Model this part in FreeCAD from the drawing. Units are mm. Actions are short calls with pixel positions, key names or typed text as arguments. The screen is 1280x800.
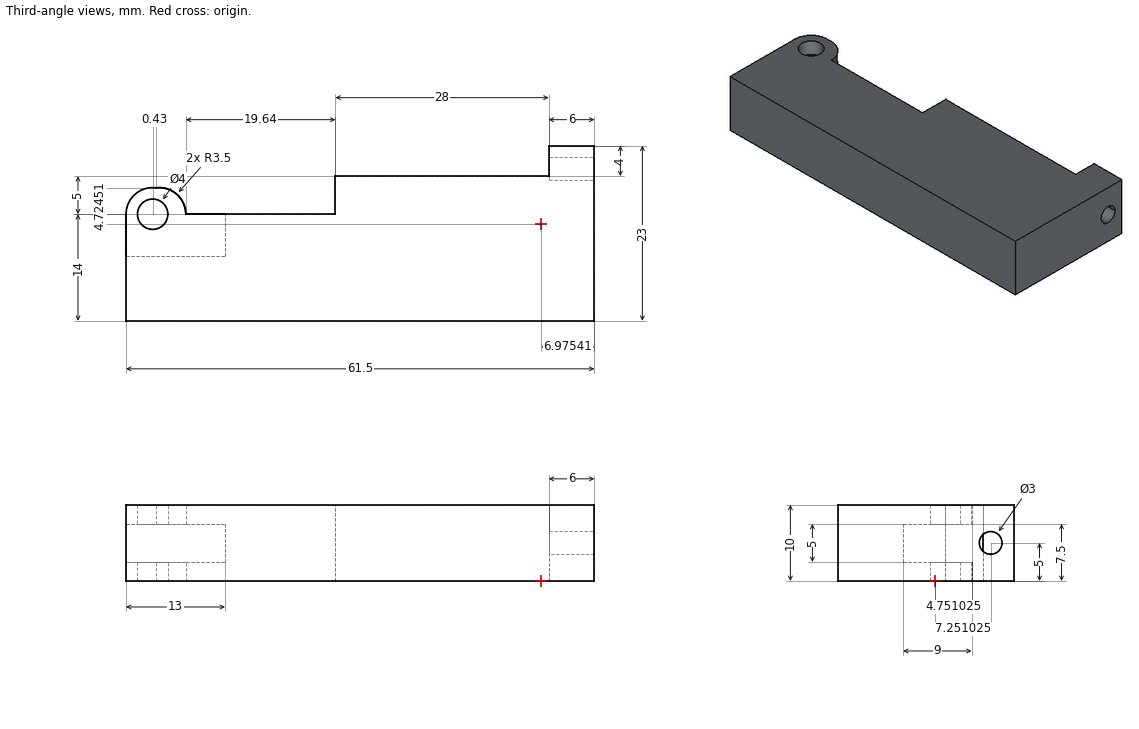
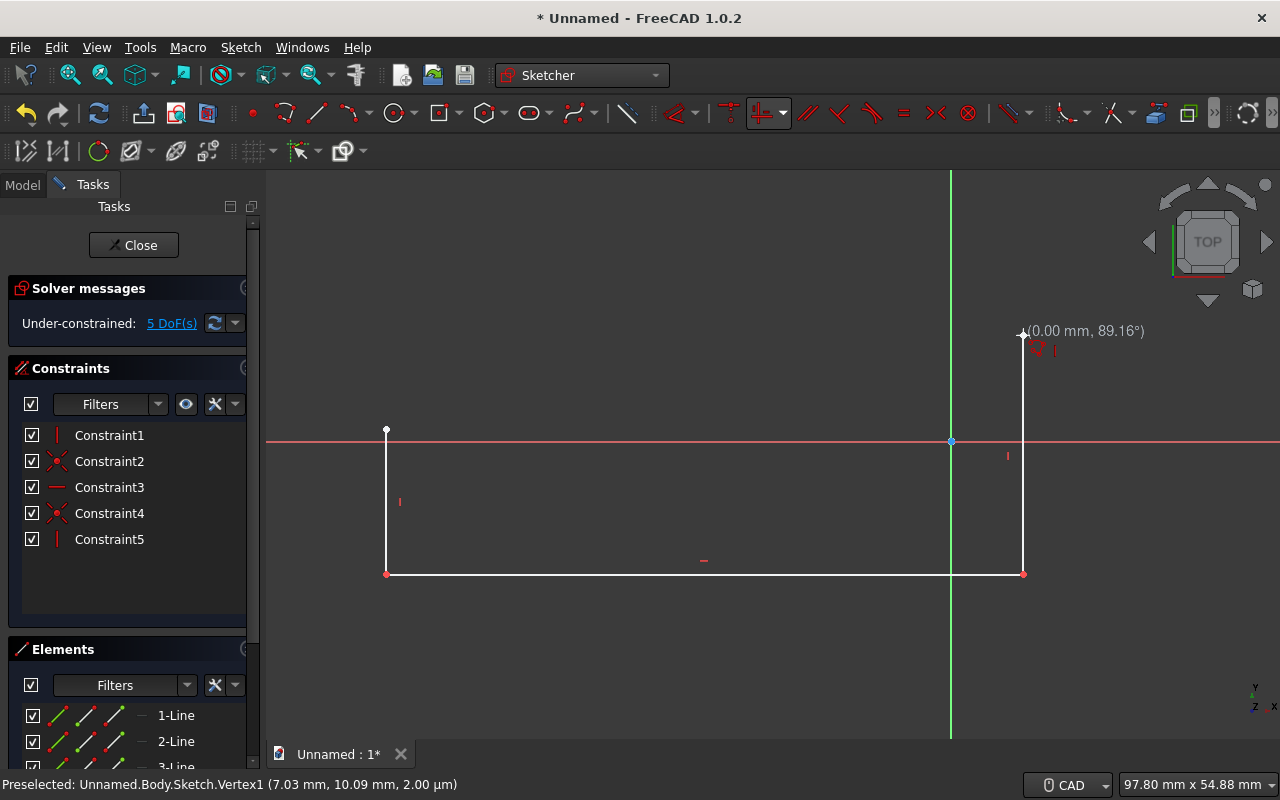
scroll(961, 335, up, 3)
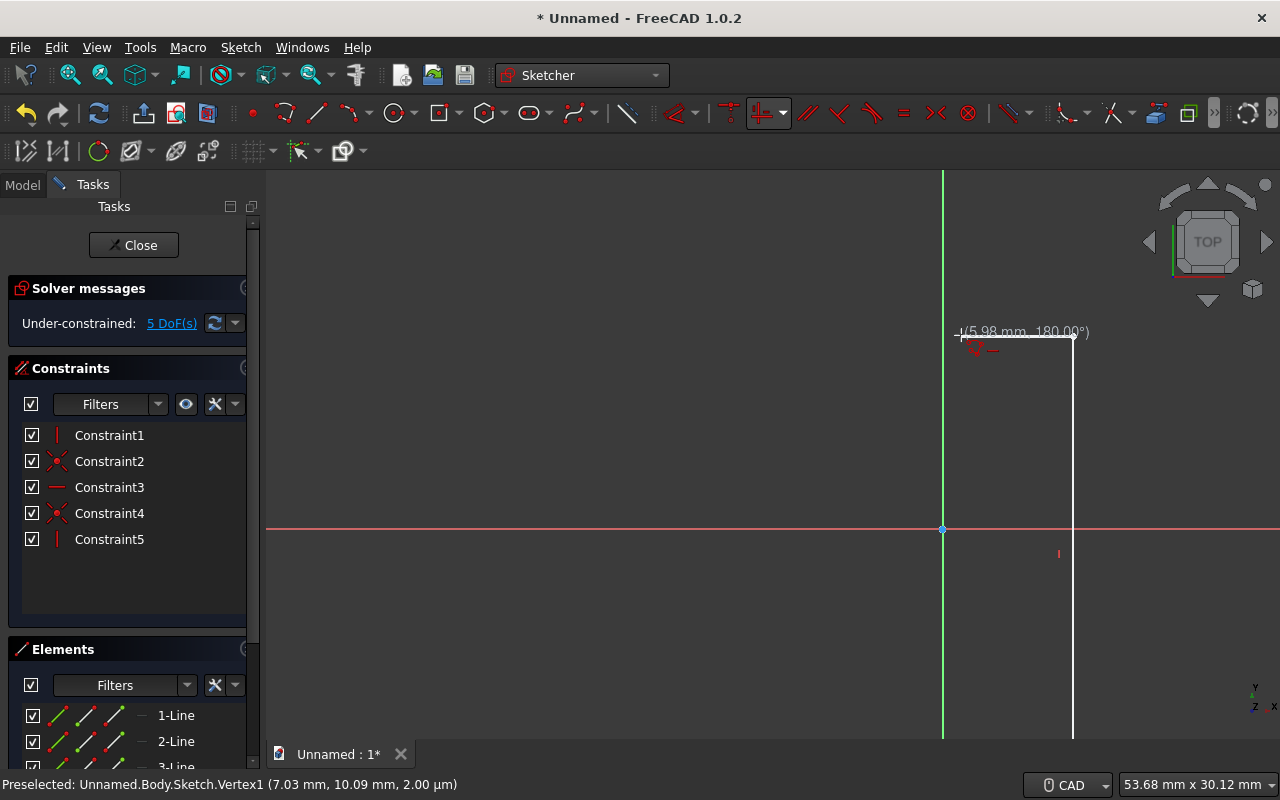
click(961, 335)
click(961, 411)
click(432, 411)
click(432, 505)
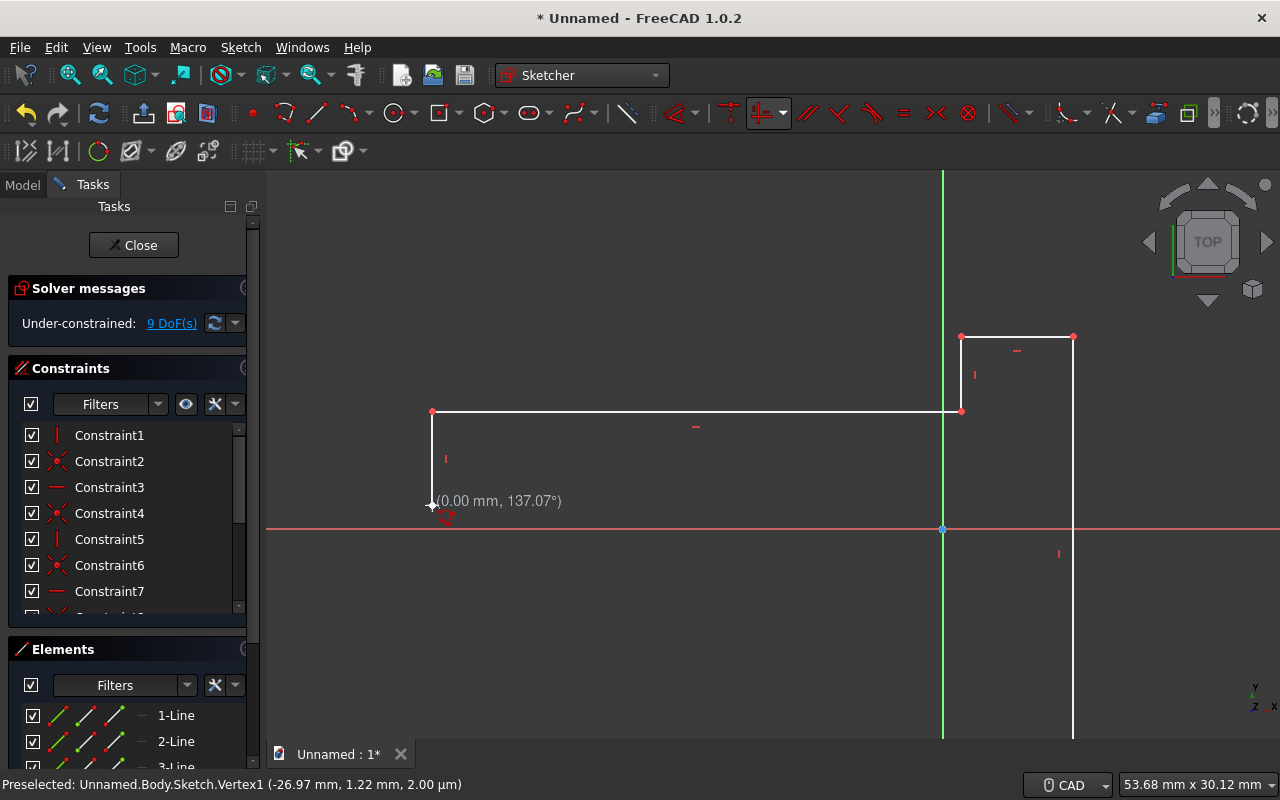
scroll(961, 335, down, 3)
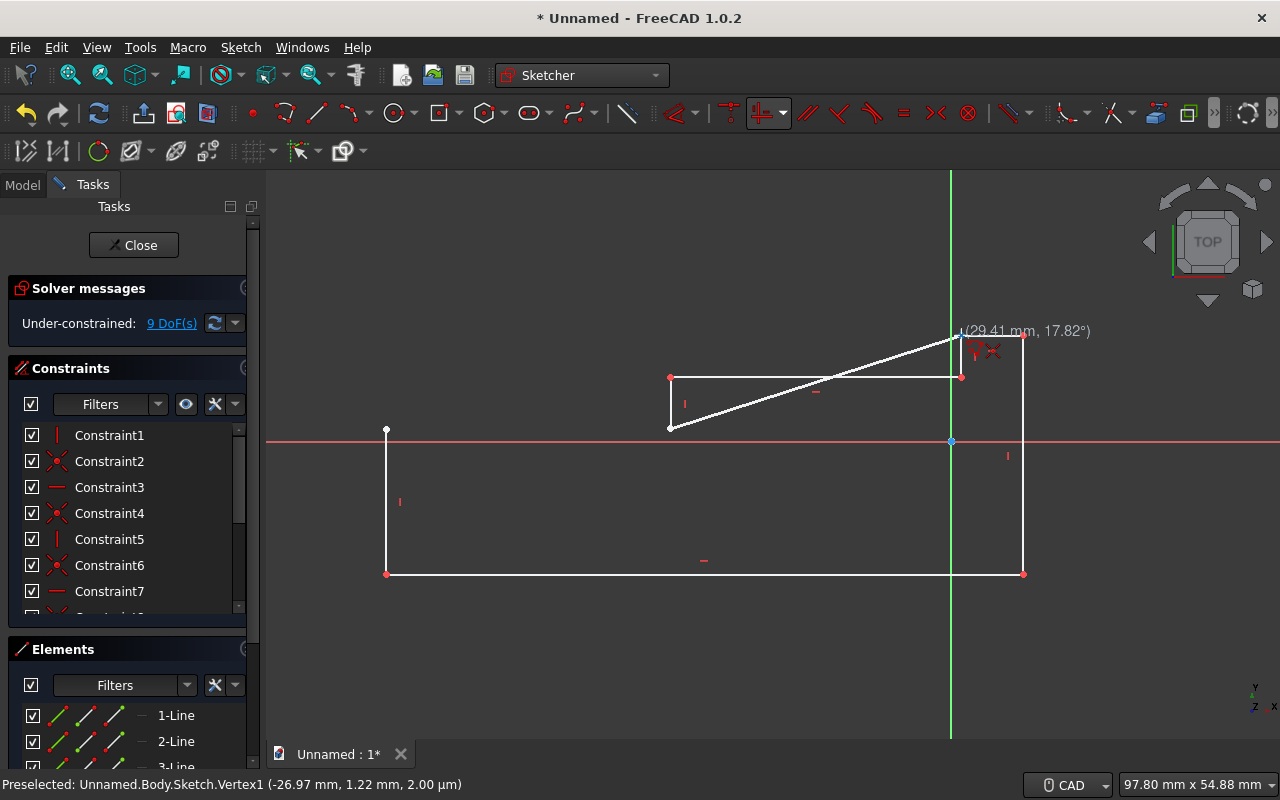
scroll(467, 429, up, 2)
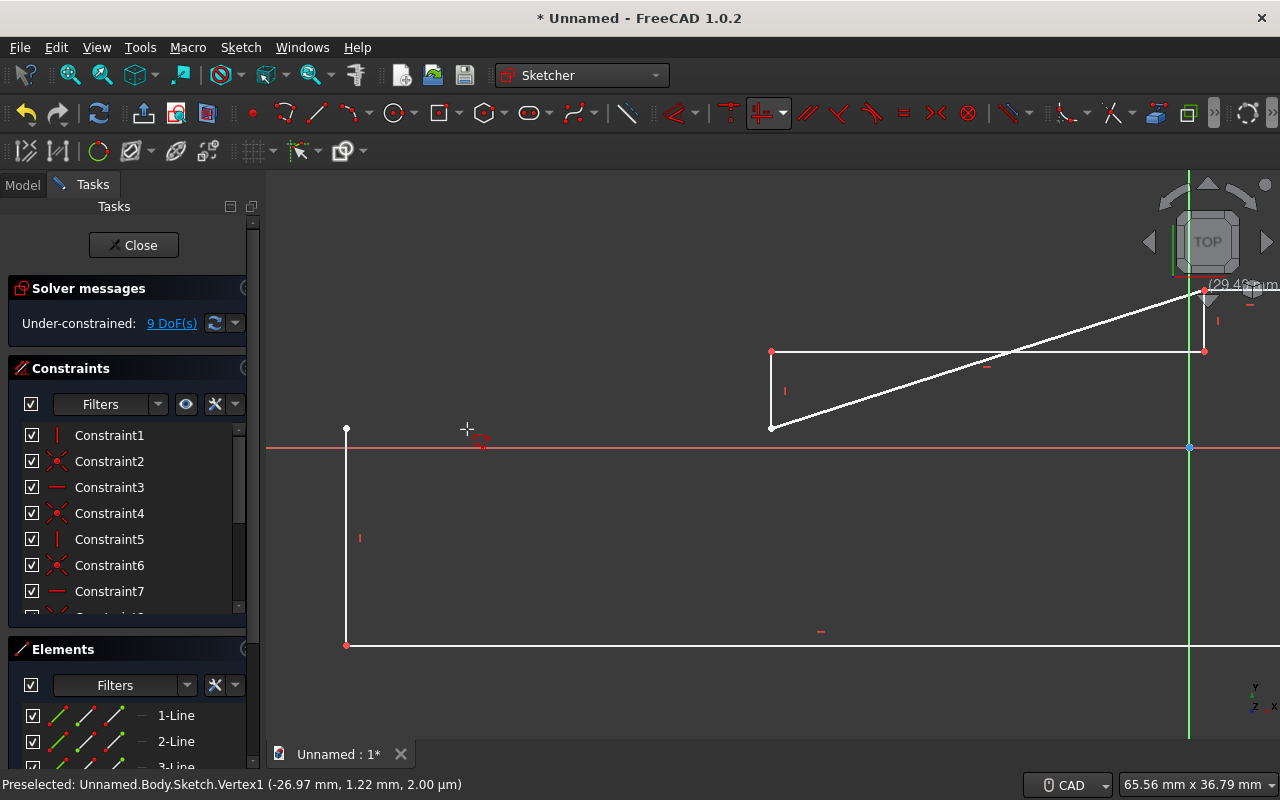
click(467, 428)
right_click(467, 428)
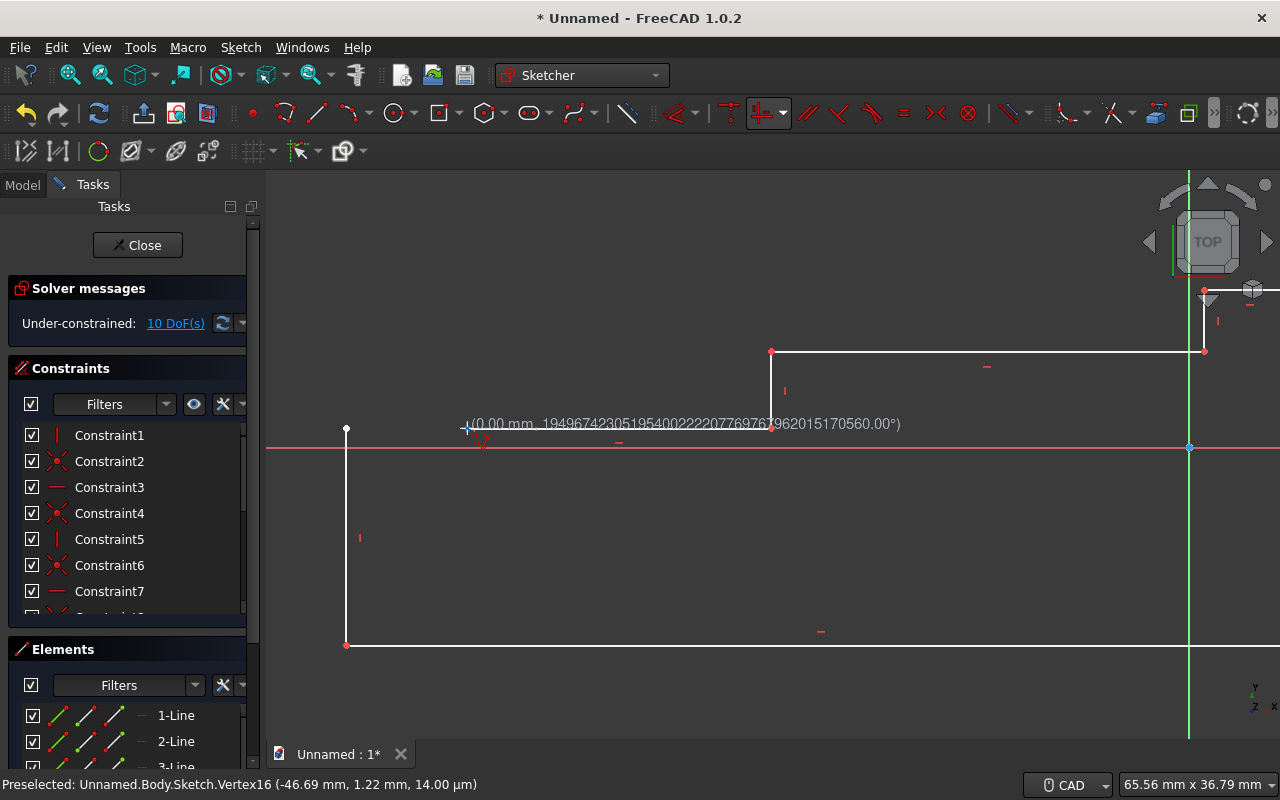
key(g)
key(3)
key(a)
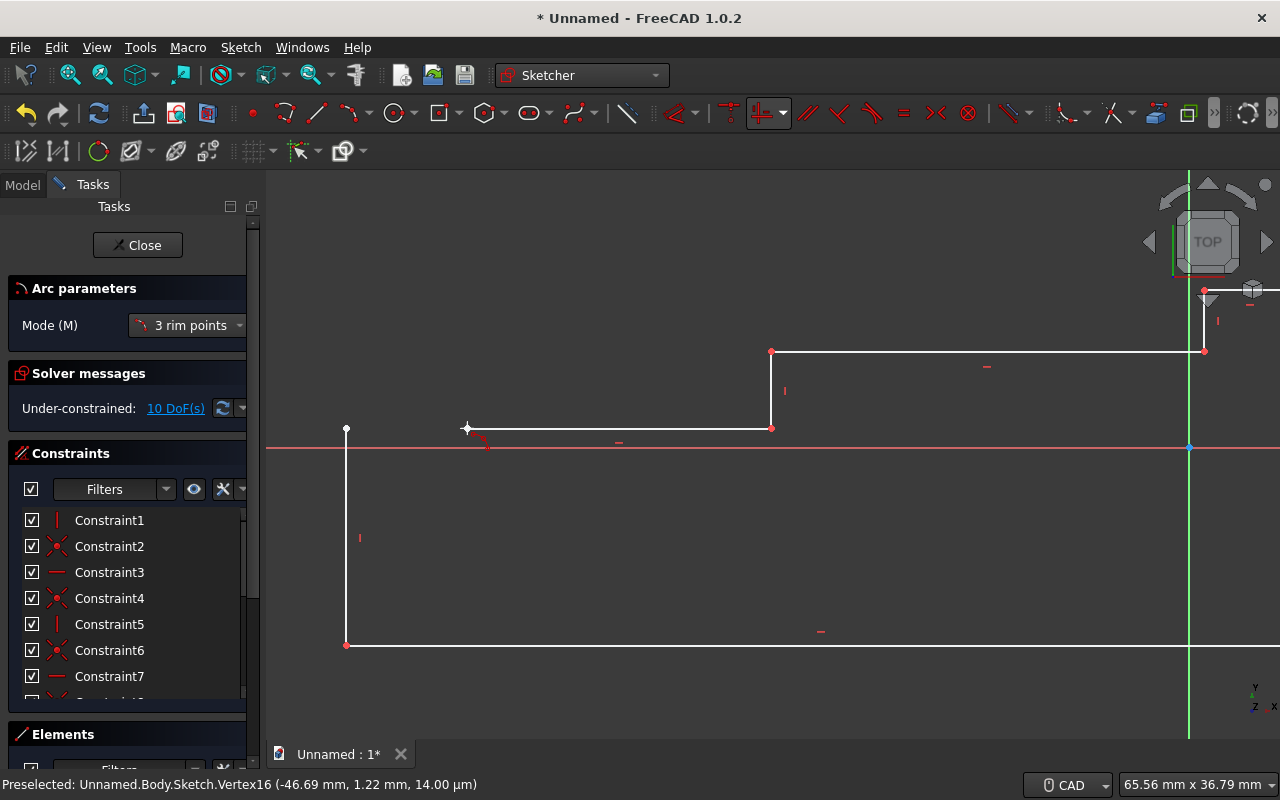
click(467, 429)
click(407, 375)
click(449, 388)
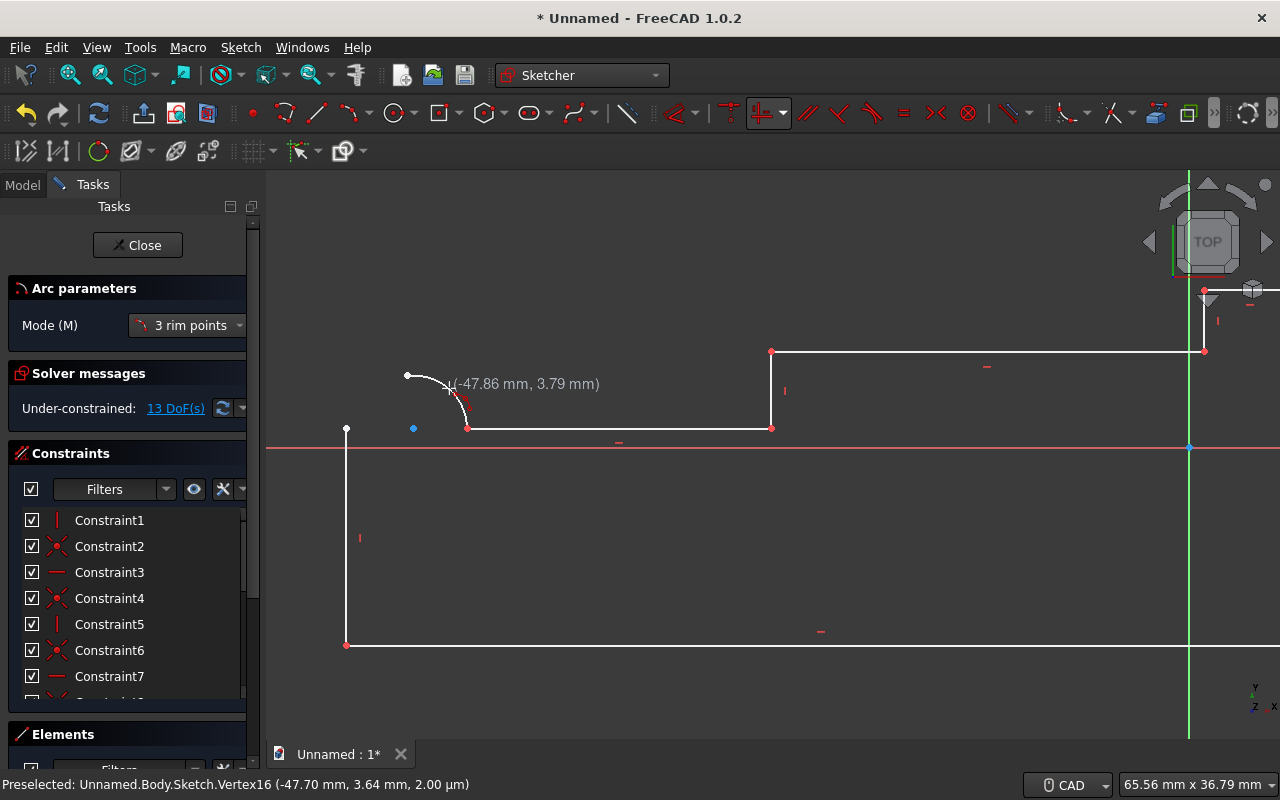
click(407, 376)
click(346, 429)
click(364, 388)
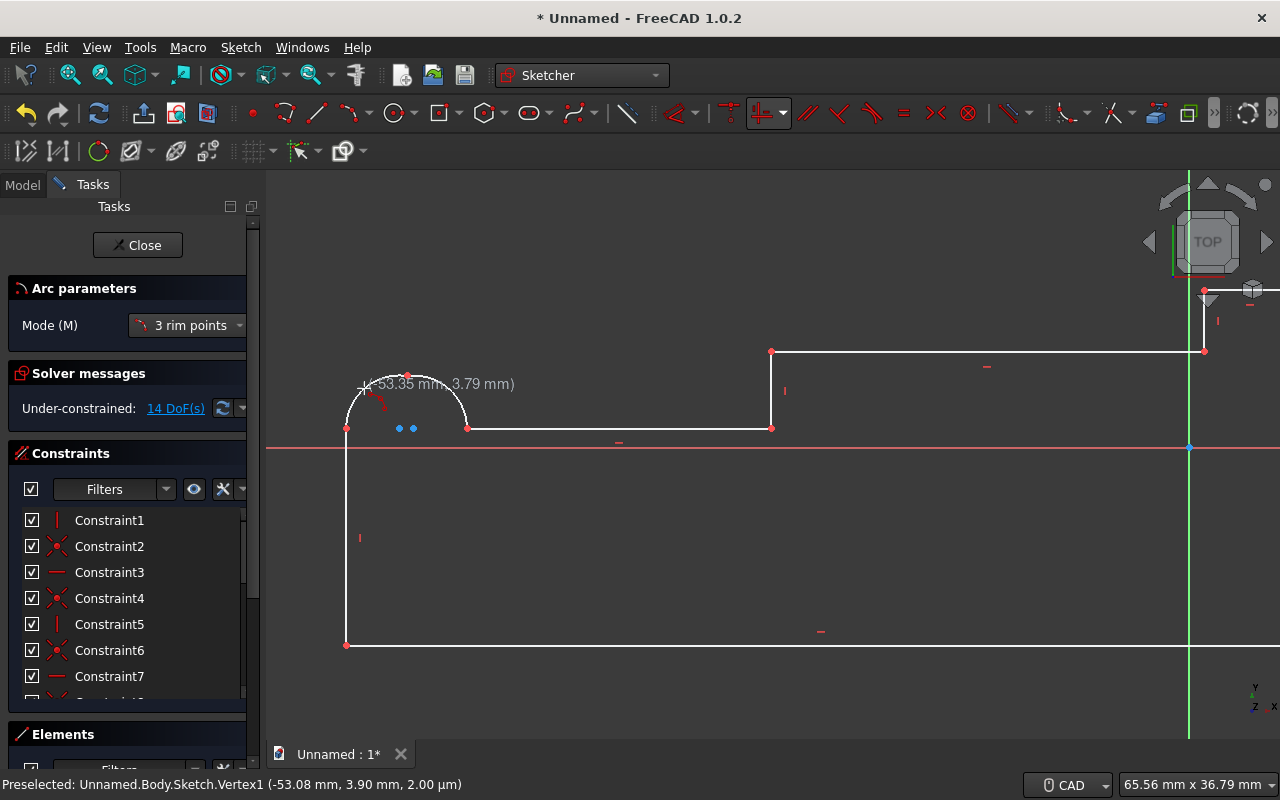
key(g)
key(c)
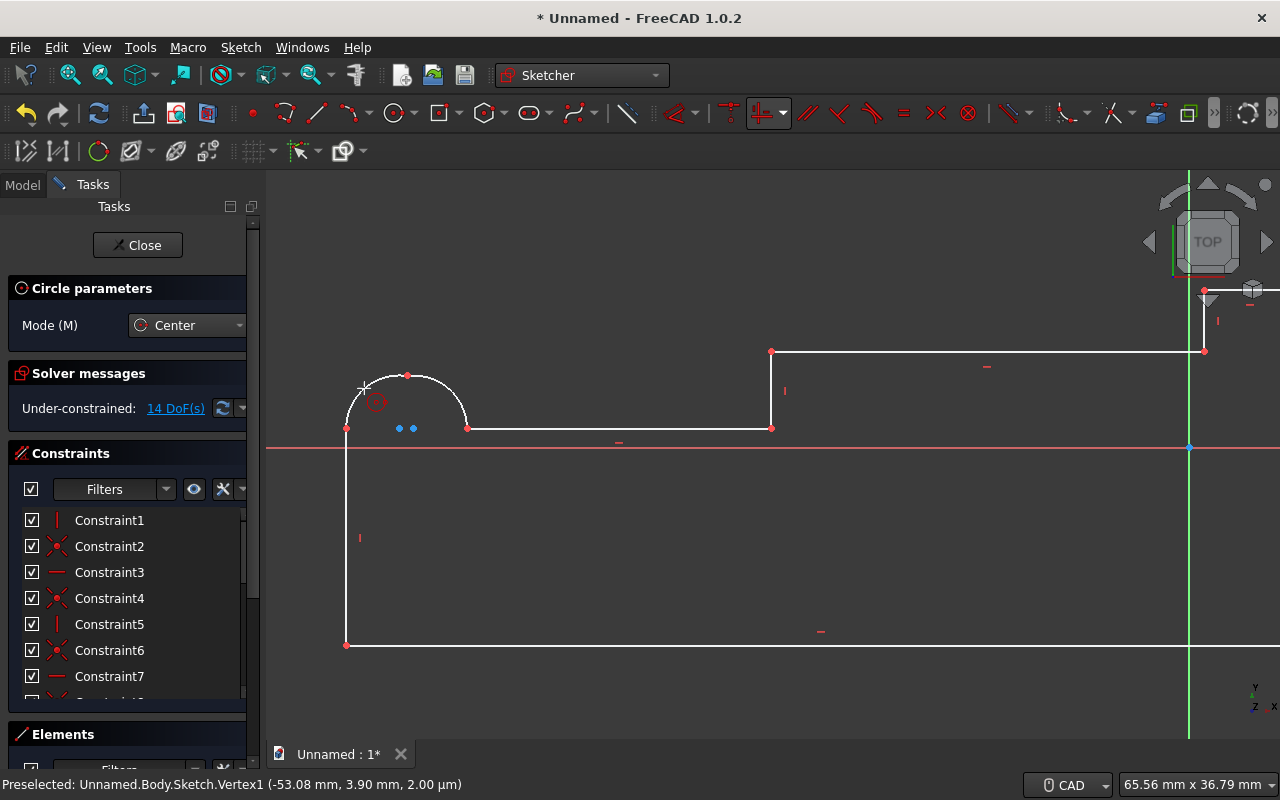
click(400, 428)
move(422, 406)